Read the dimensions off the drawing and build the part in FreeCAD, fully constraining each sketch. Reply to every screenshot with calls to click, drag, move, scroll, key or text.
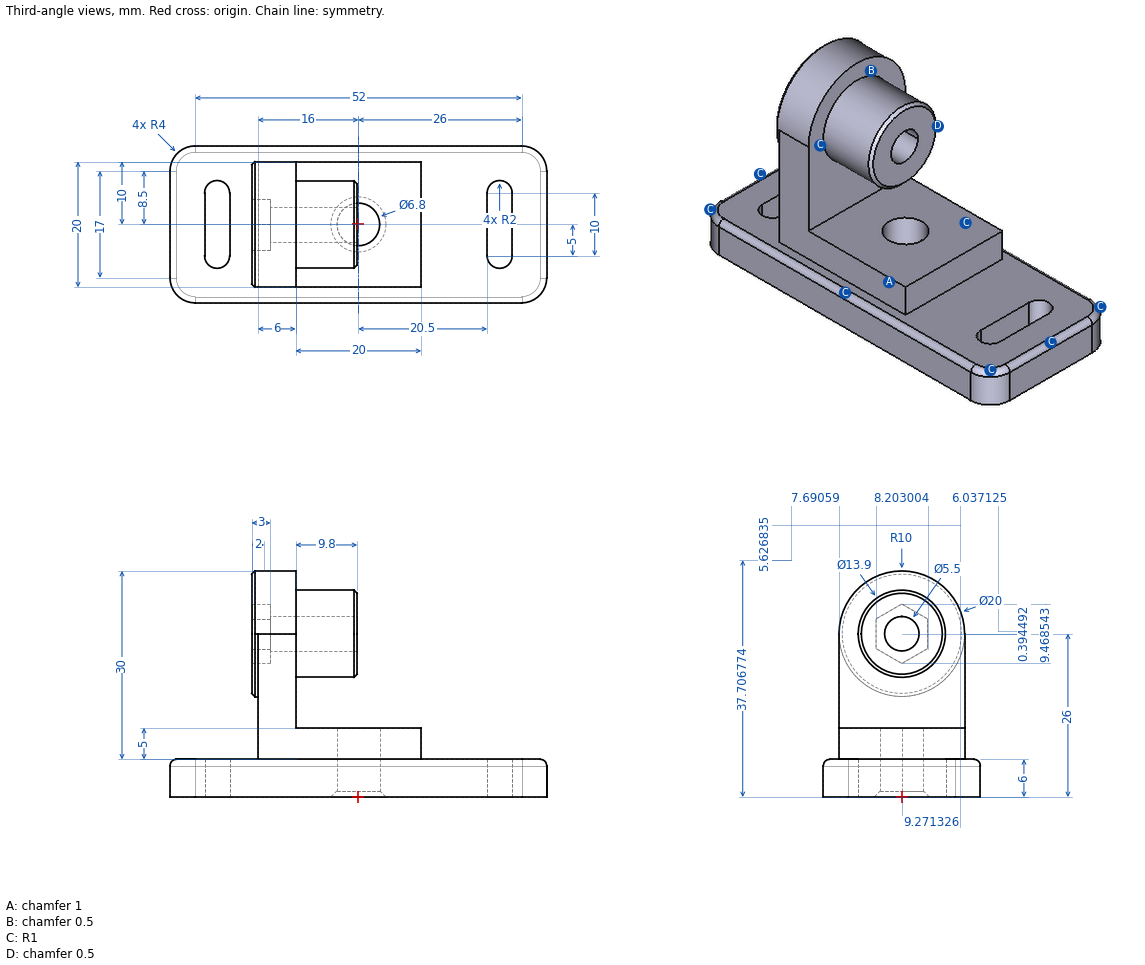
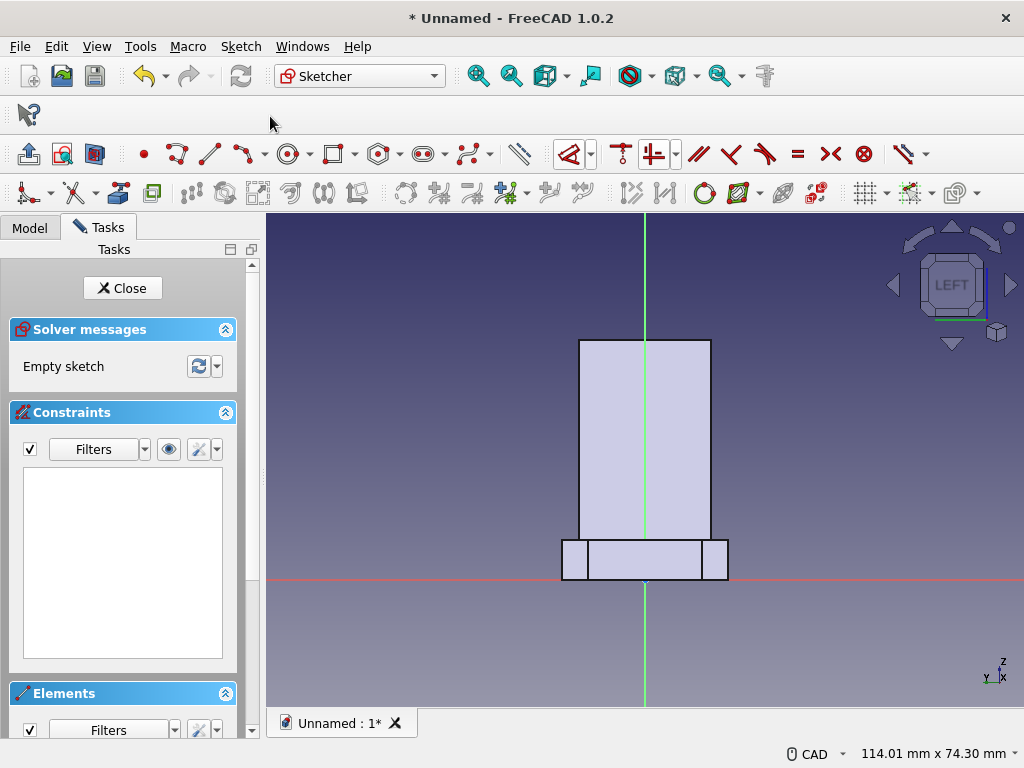
click(177, 154)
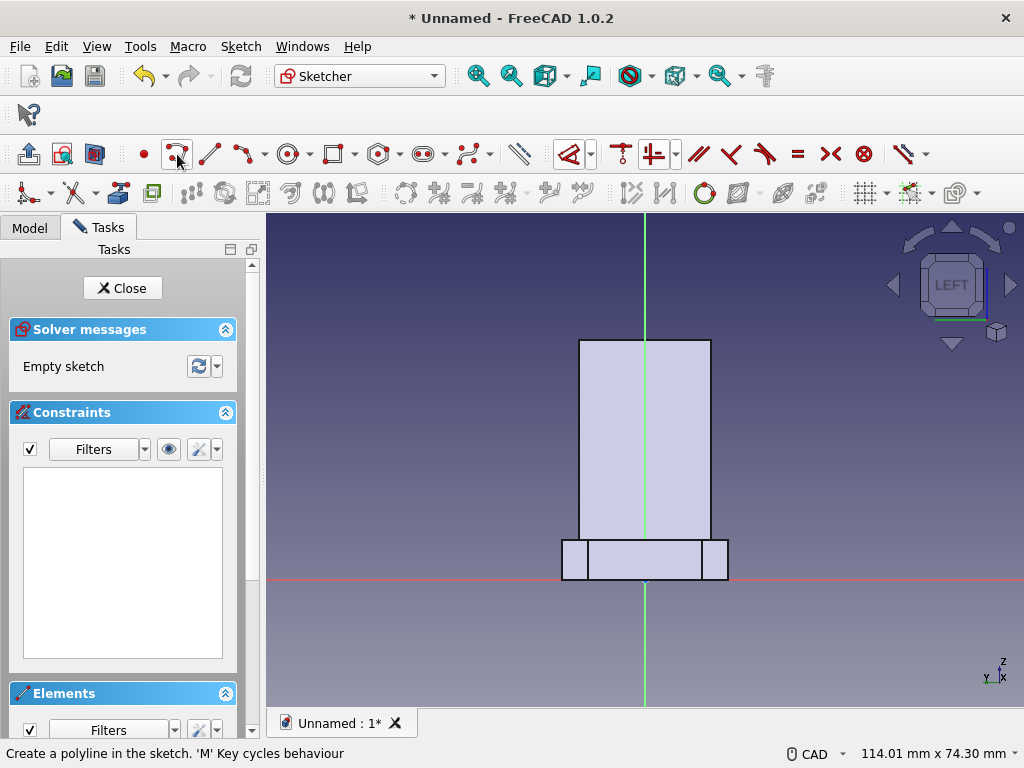
click(711, 407)
click(763, 329)
click(583, 292)
click(543, 404)
click(579, 407)
right_click(579, 407)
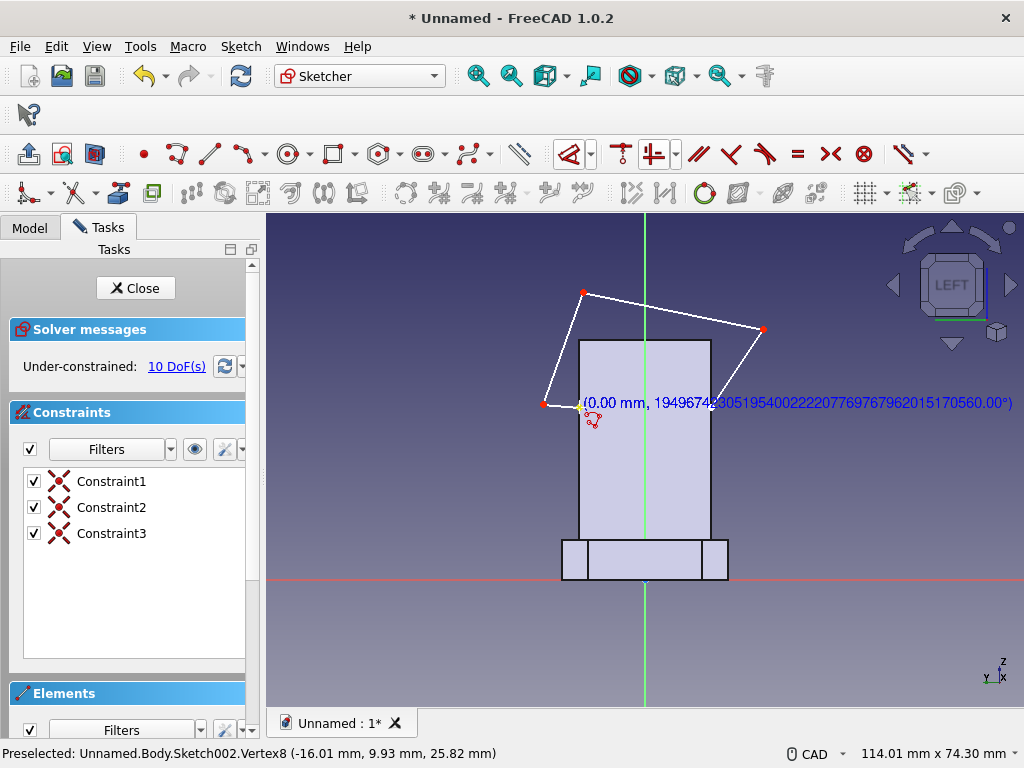
key(g)
key(3)
key(a)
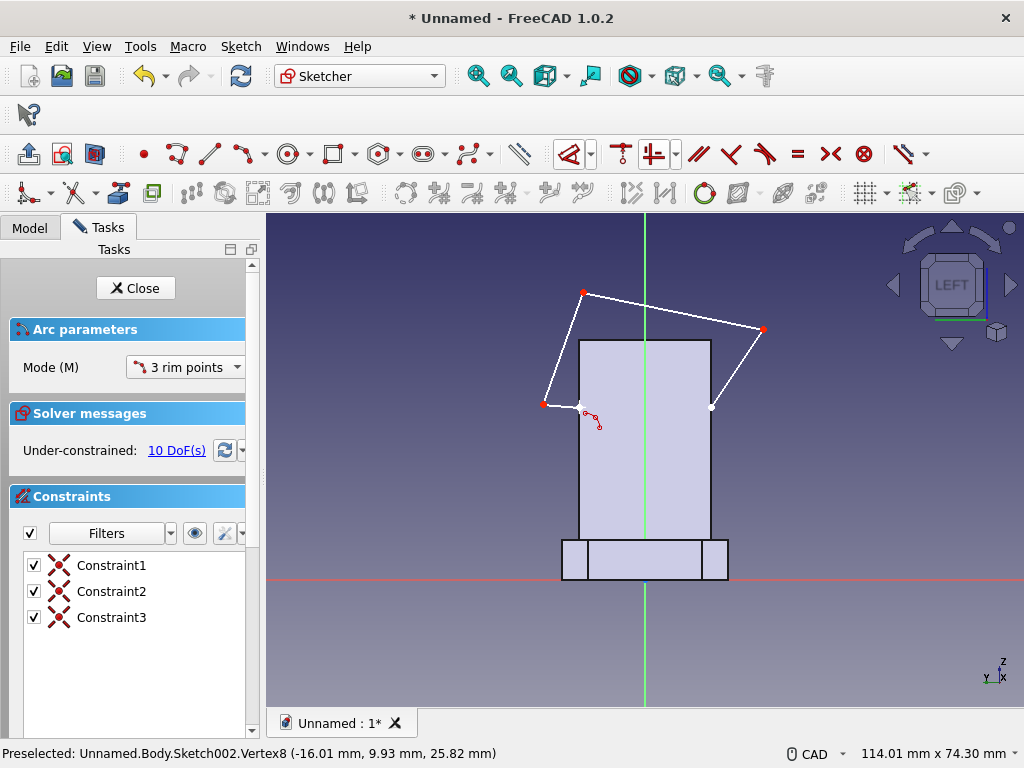
click(579, 408)
click(711, 408)
click(666, 344)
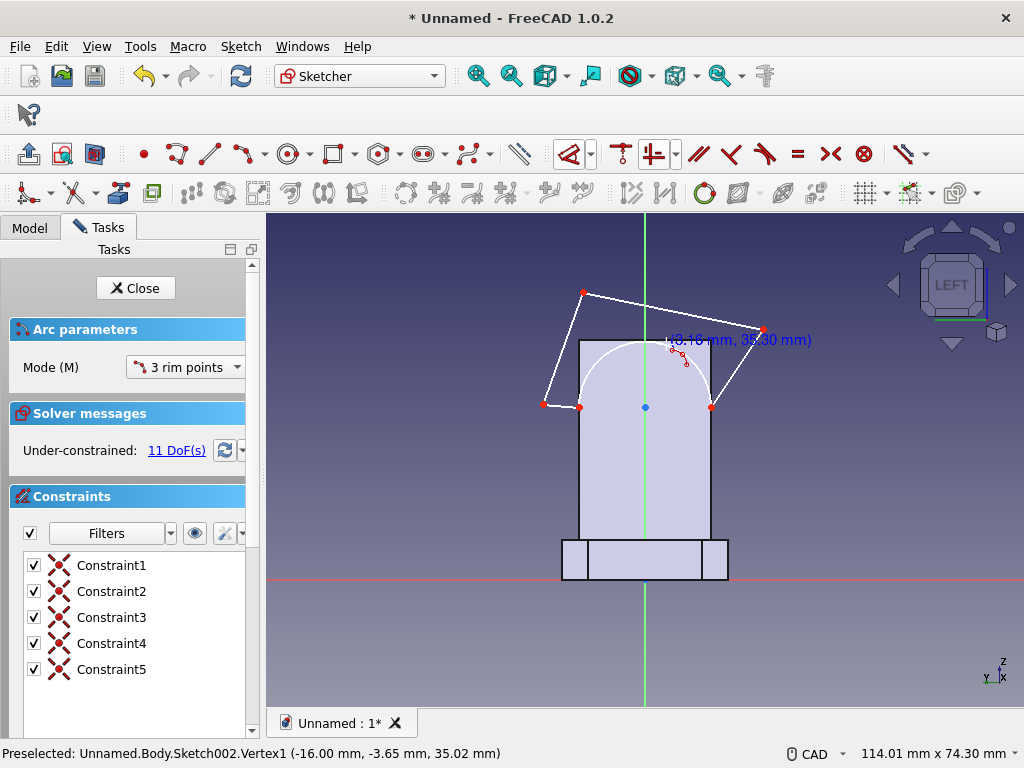
click(288, 154)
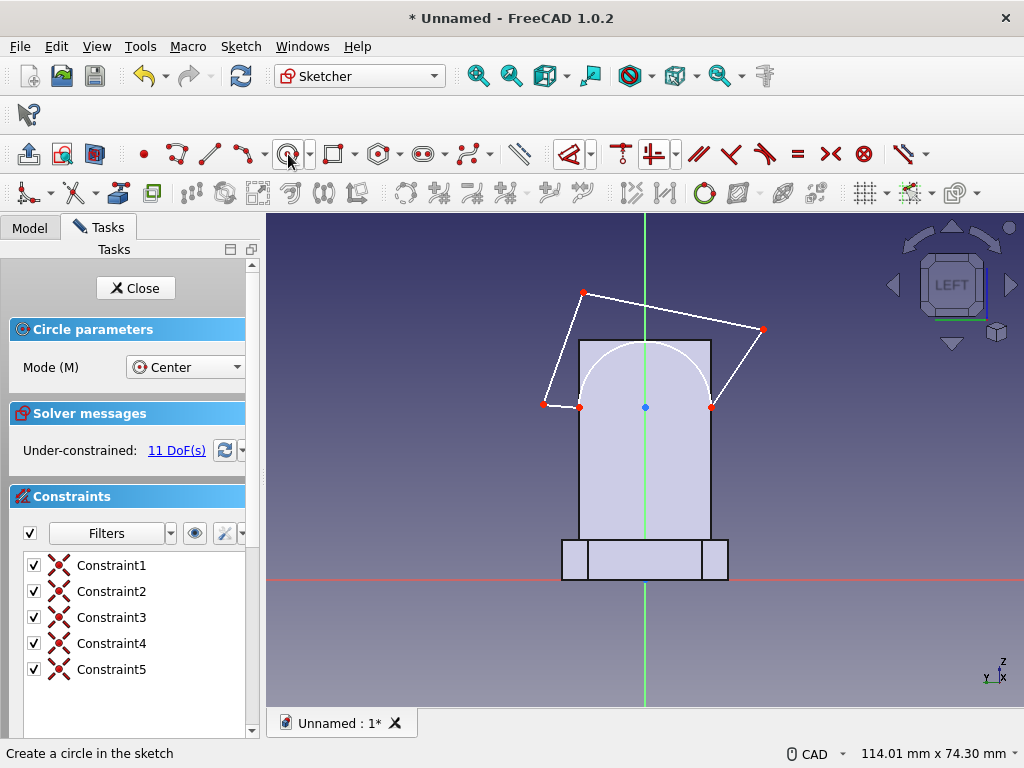
scroll(645, 407, up, 2)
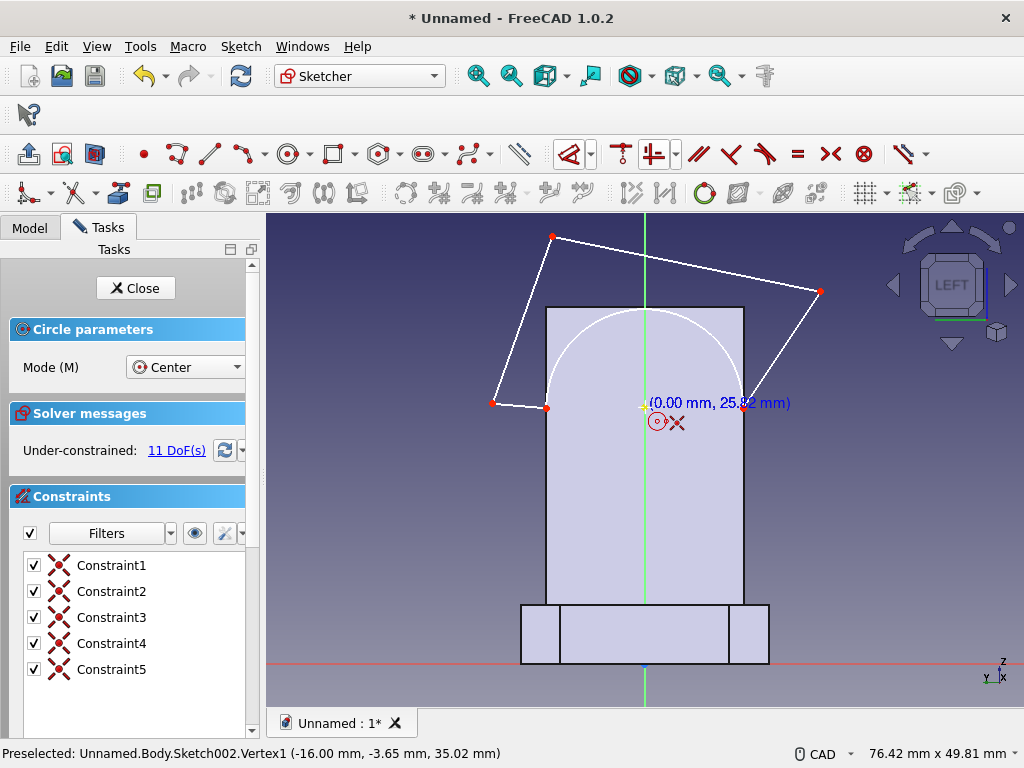
click(645, 407)
move(664, 387)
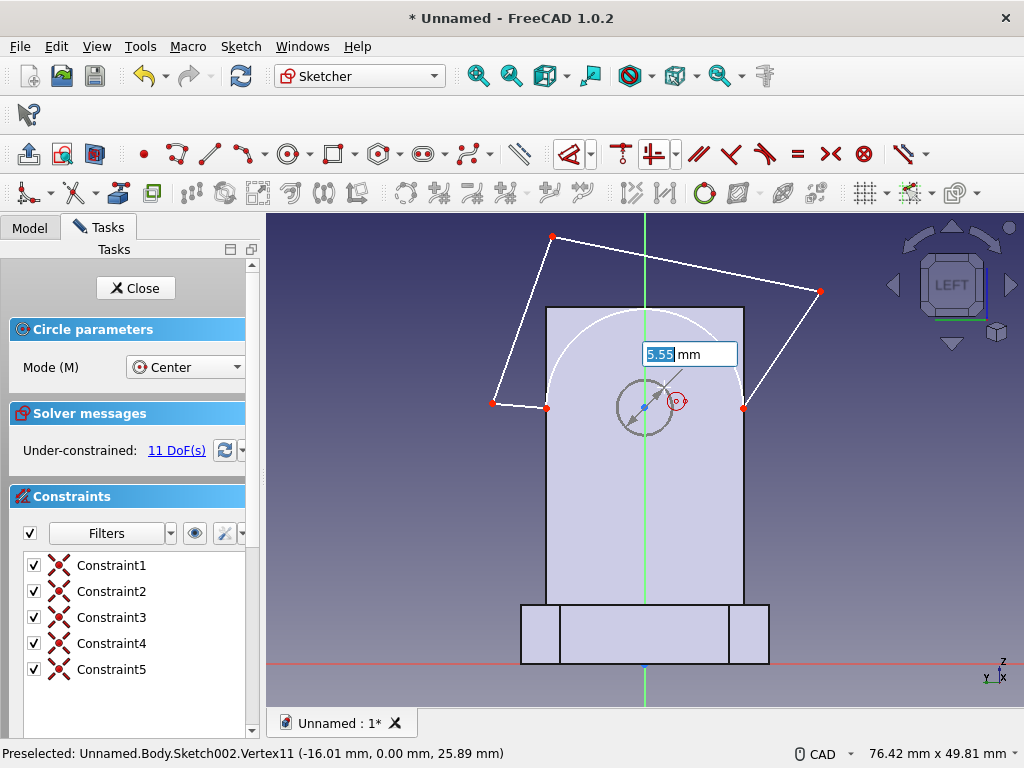
text(5.5)
key(Return)
key(Escape)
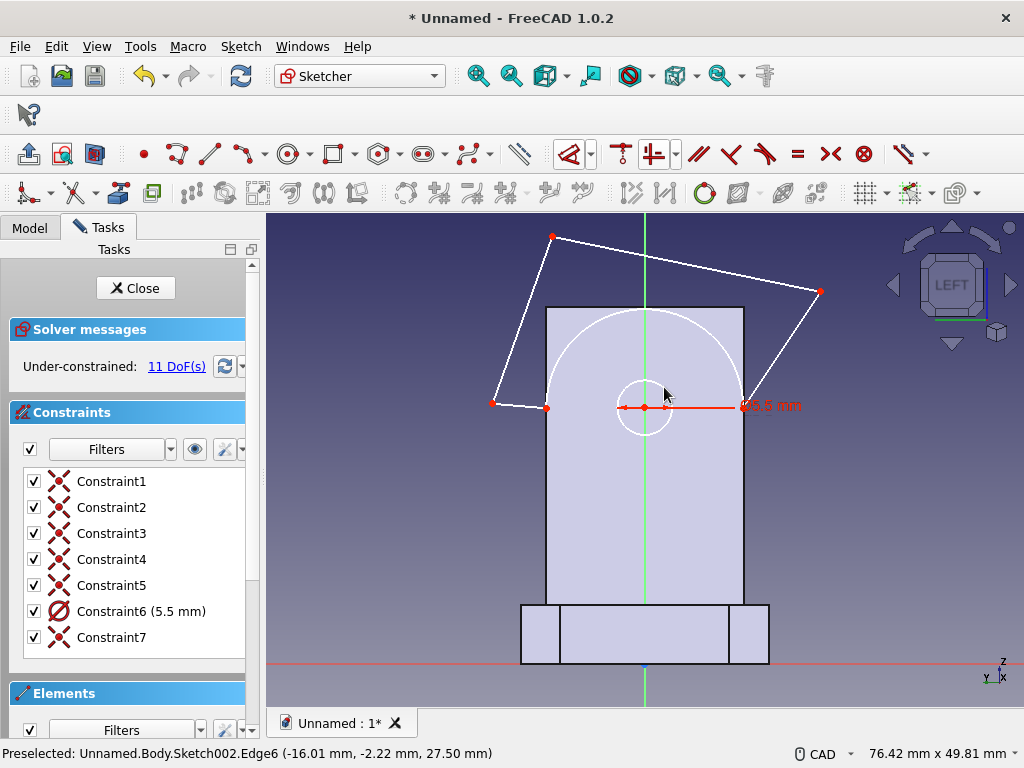
click(645, 408)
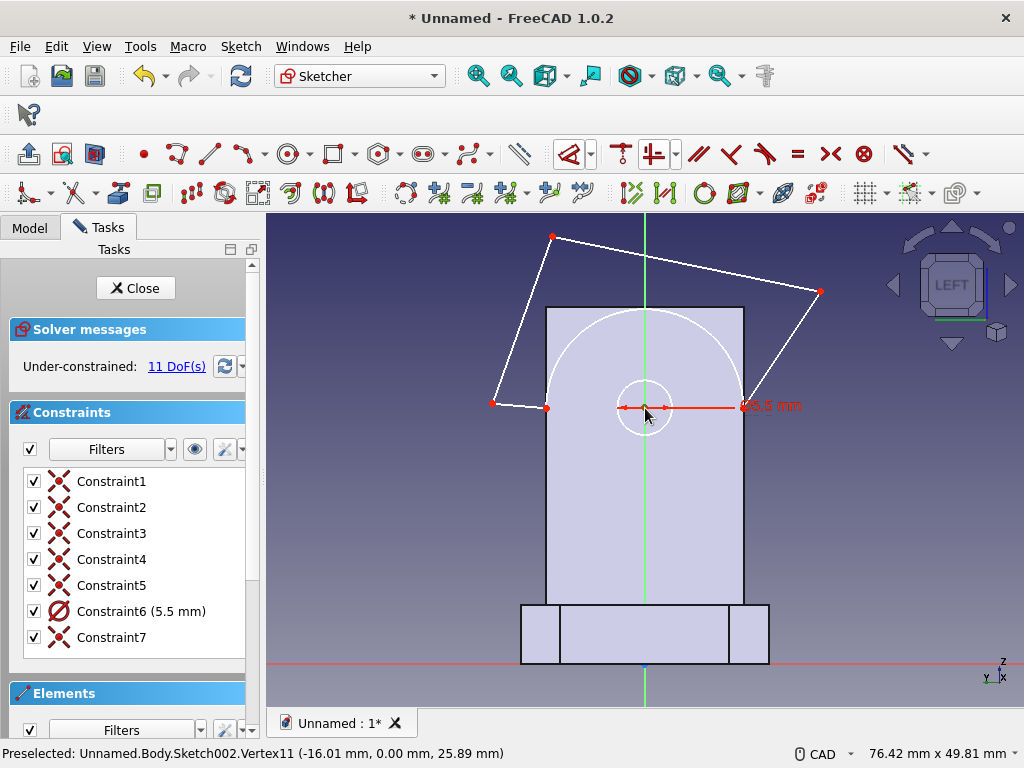
click(645, 616)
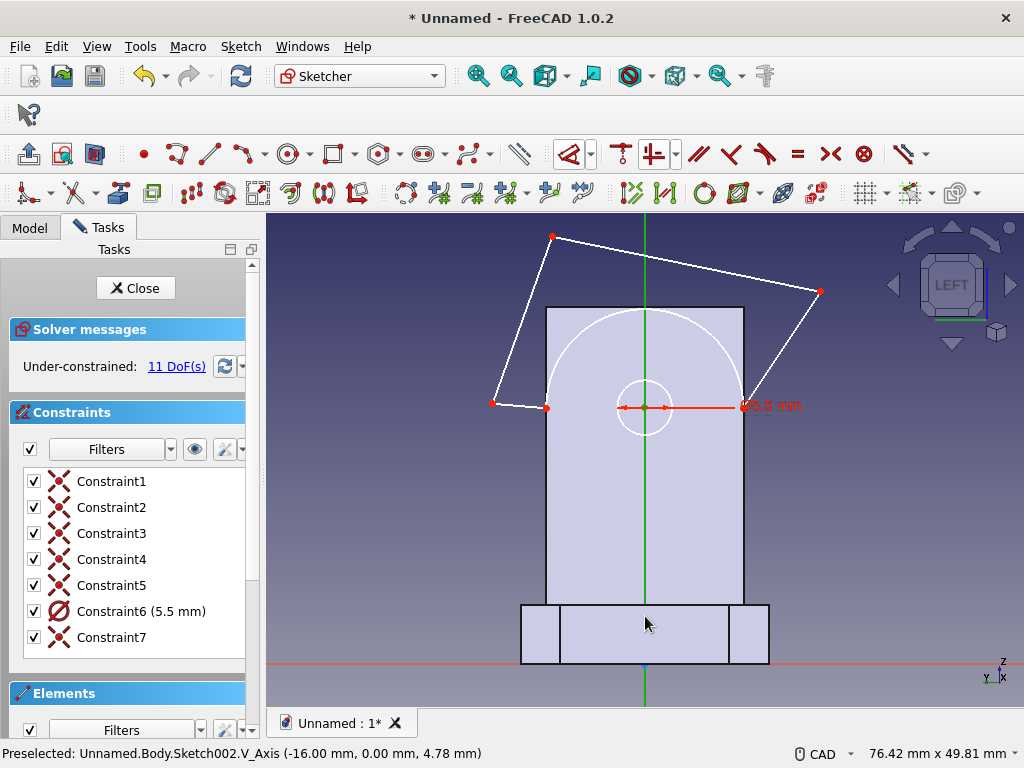
click(621, 154)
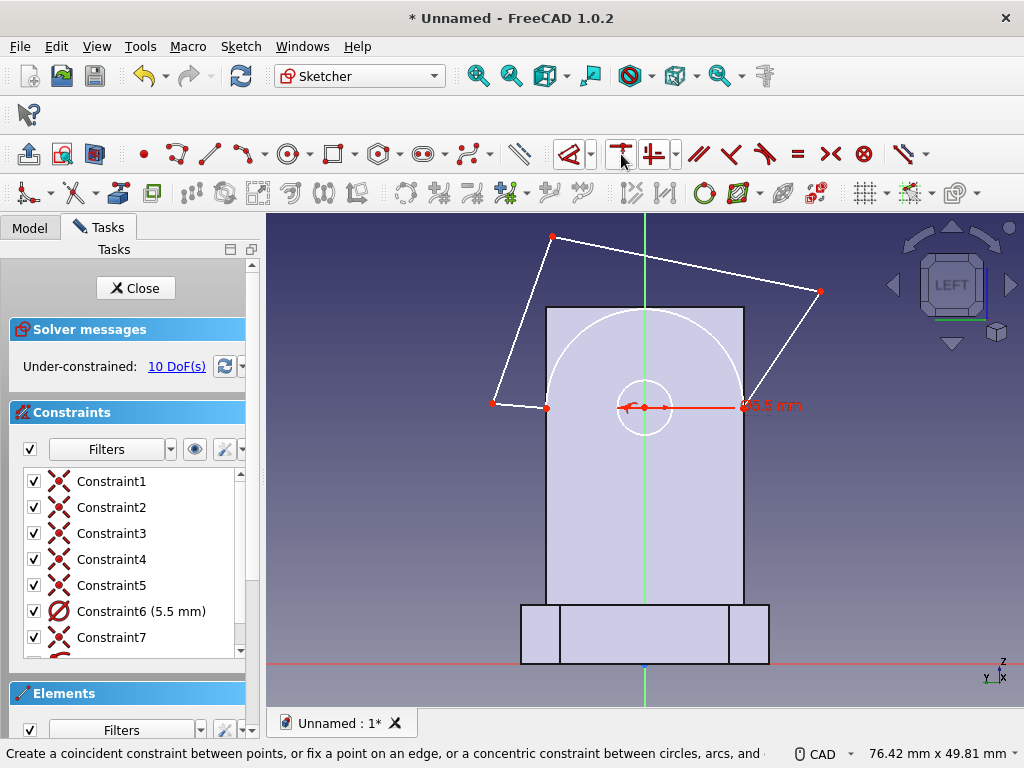
click(703, 328)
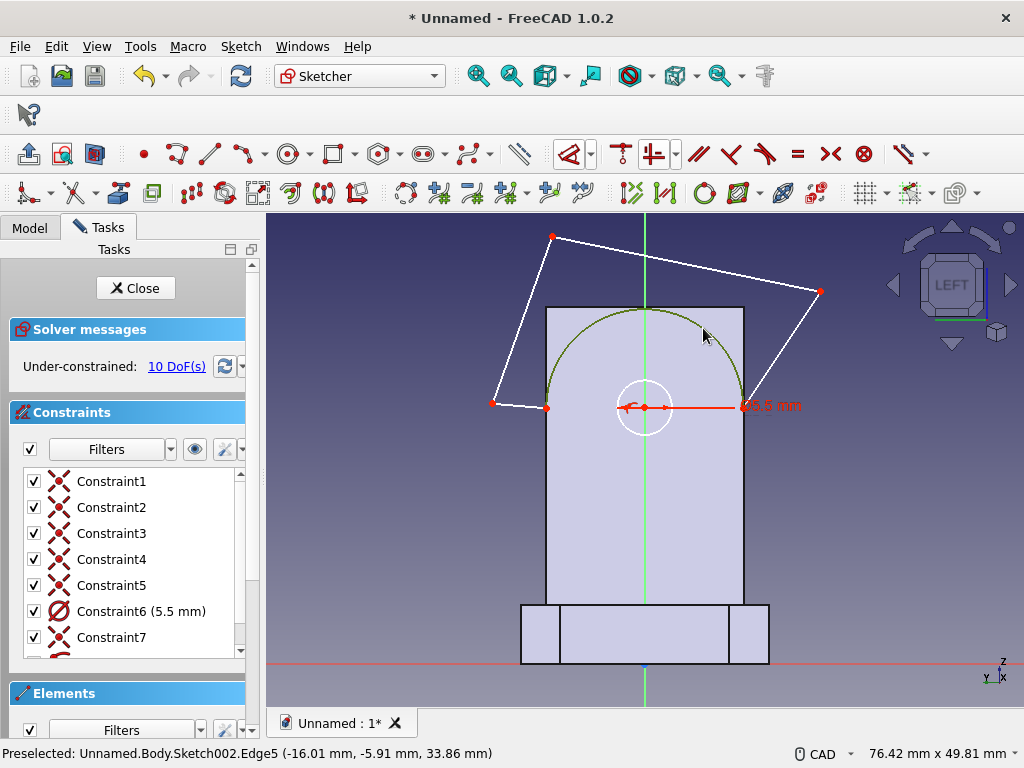
click(590, 154)